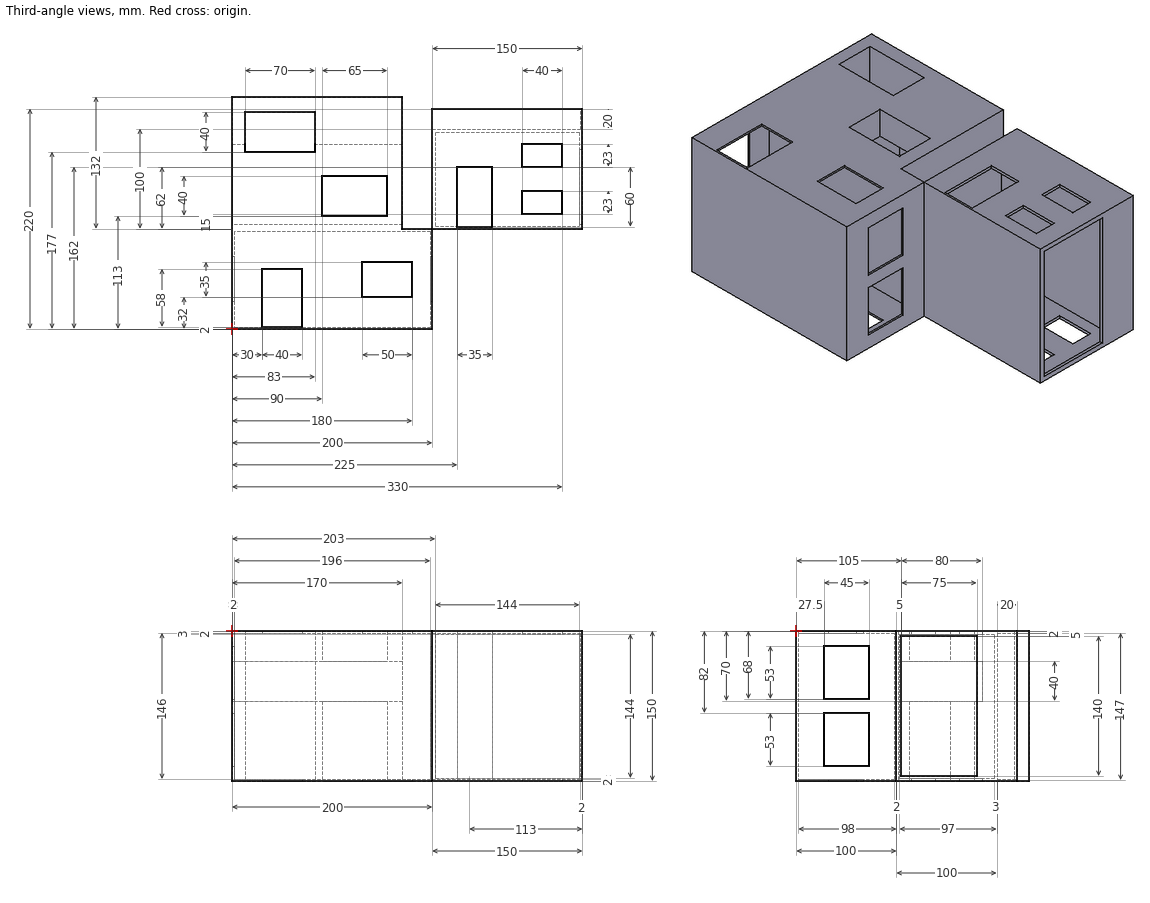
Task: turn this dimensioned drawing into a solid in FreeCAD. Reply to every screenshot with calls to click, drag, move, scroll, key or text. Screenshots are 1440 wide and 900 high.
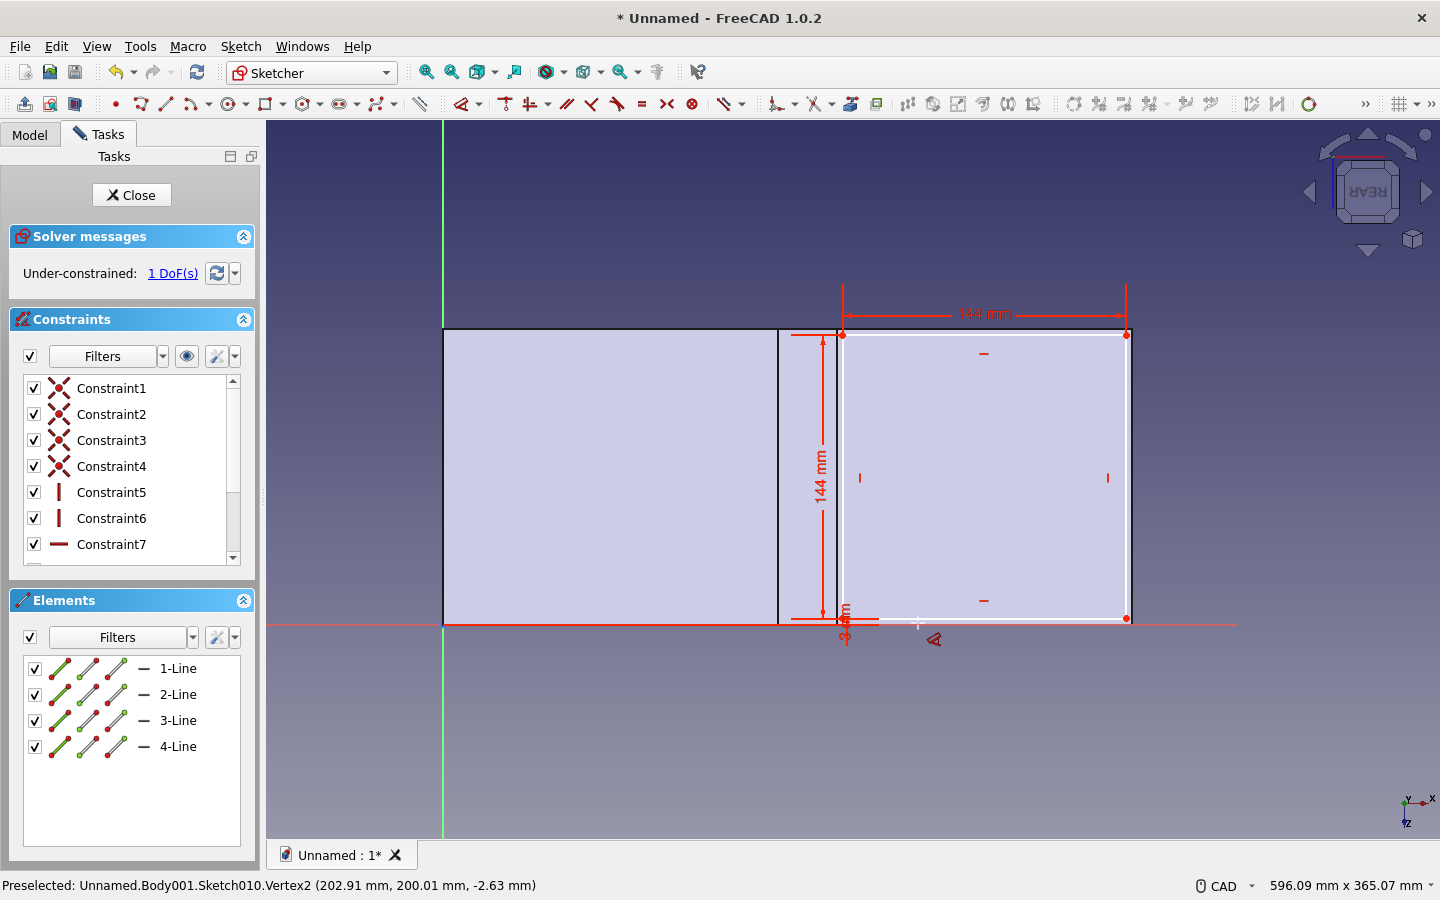
click(843, 335)
click(643, 659)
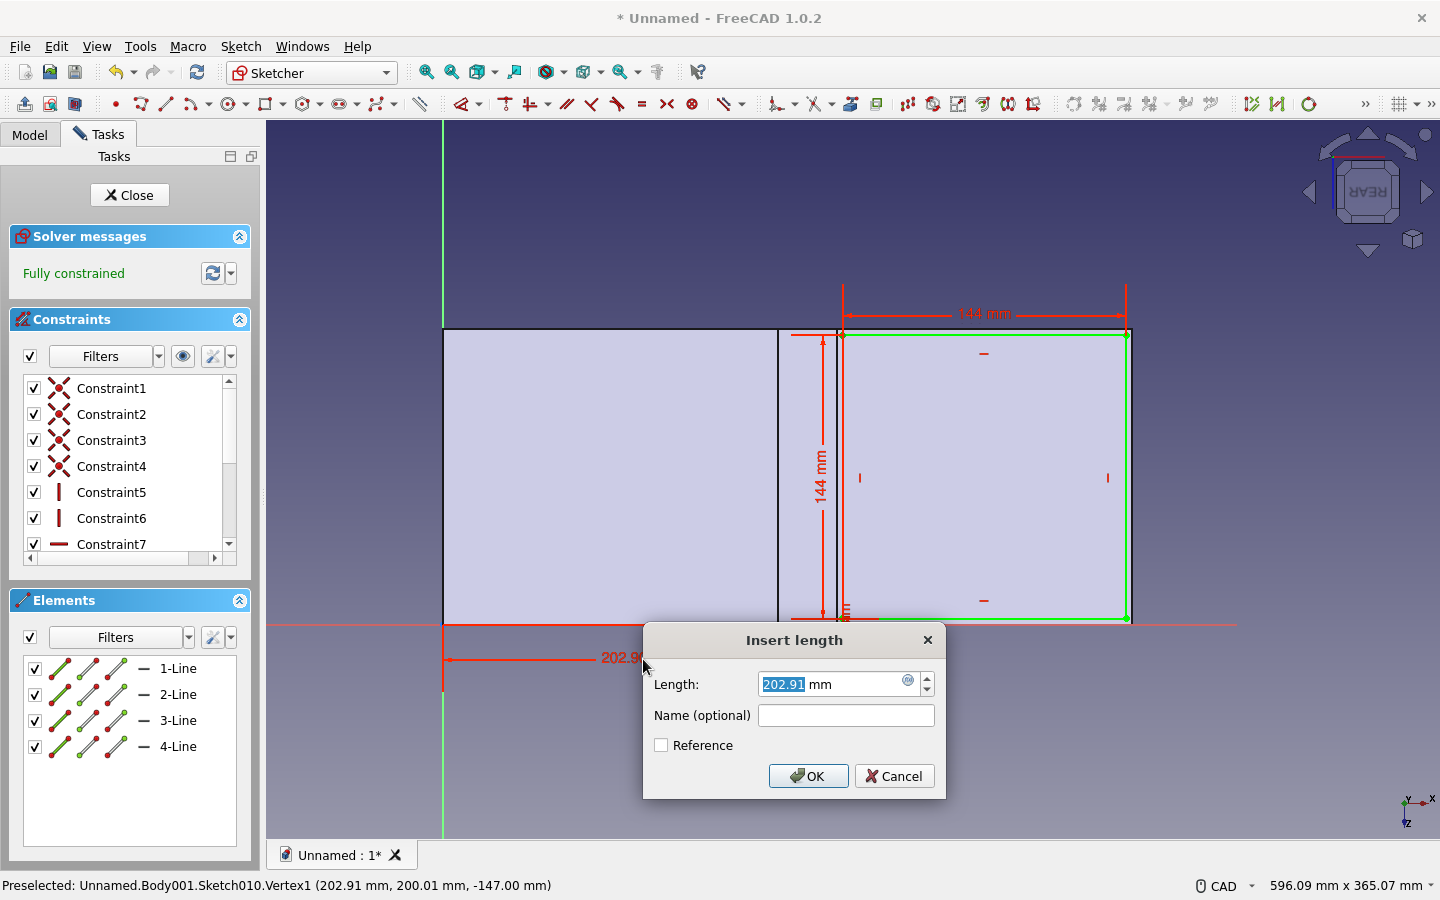
text(203)
key(Return)
key(Escape)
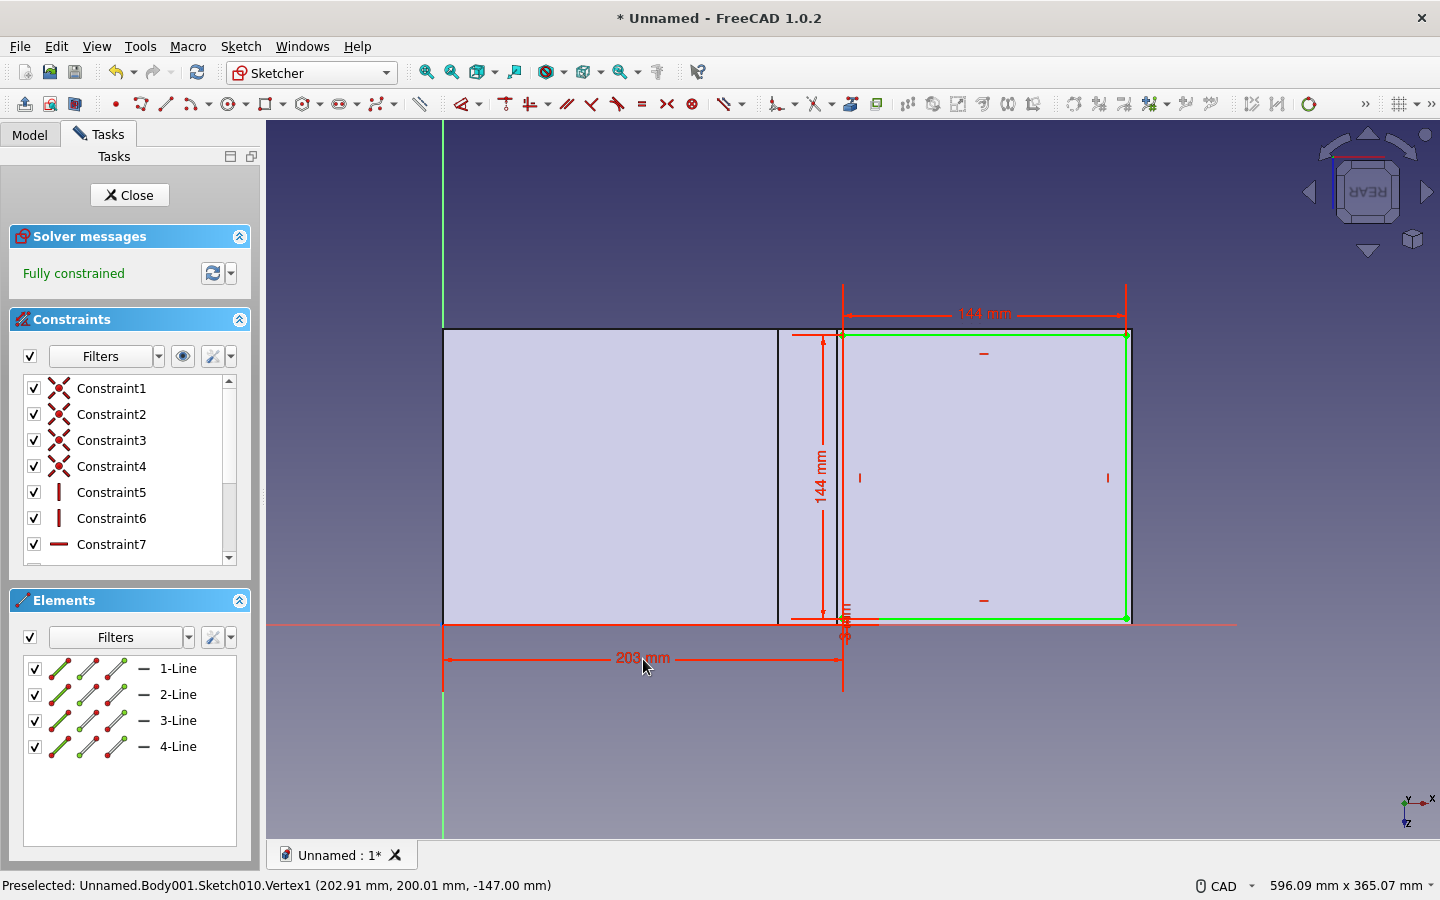
click(130, 195)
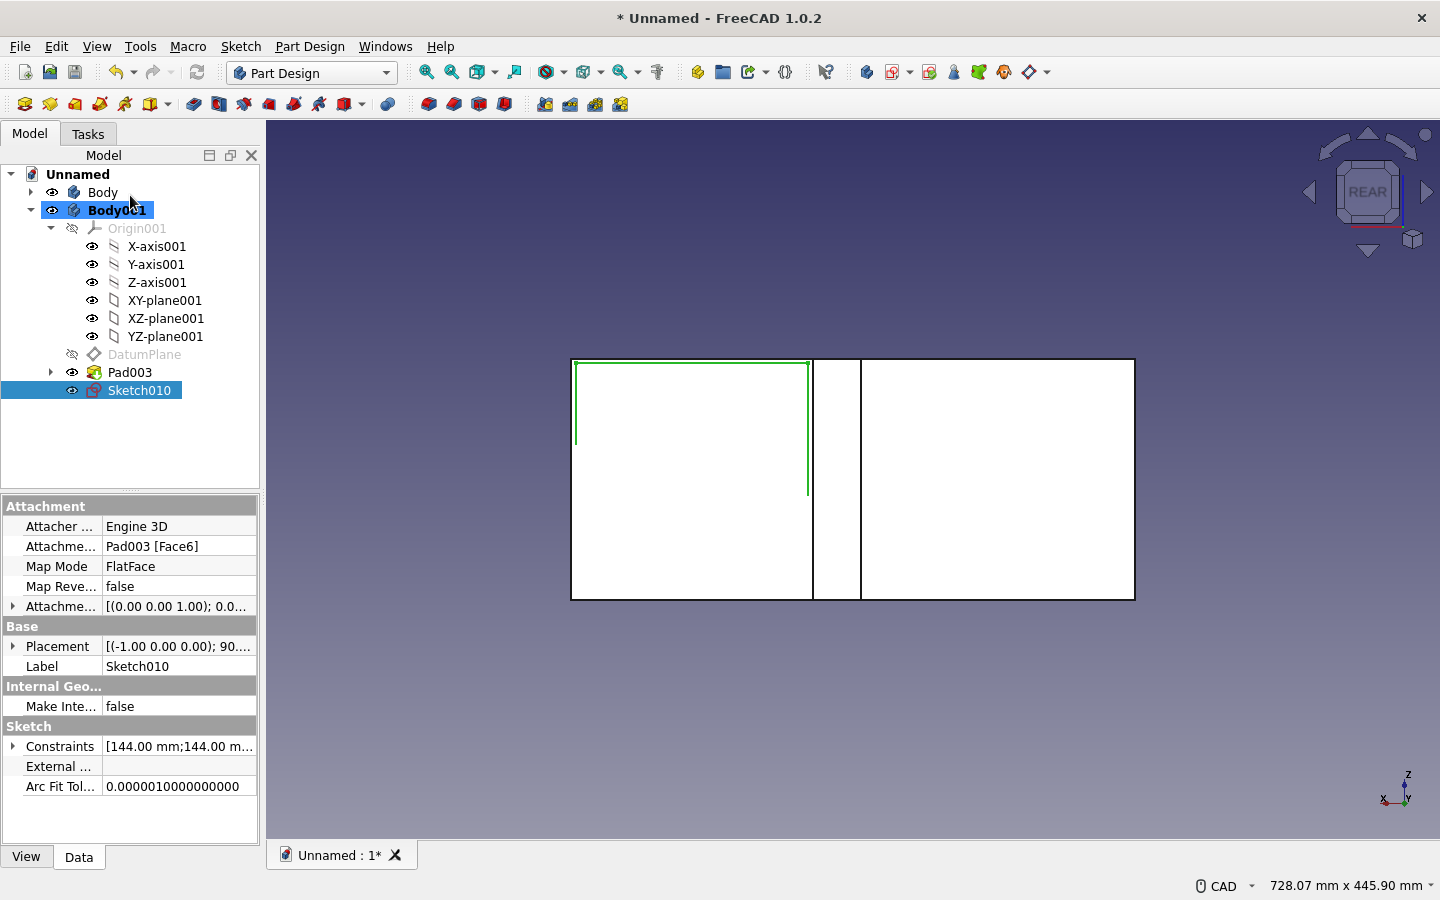
click(194, 104)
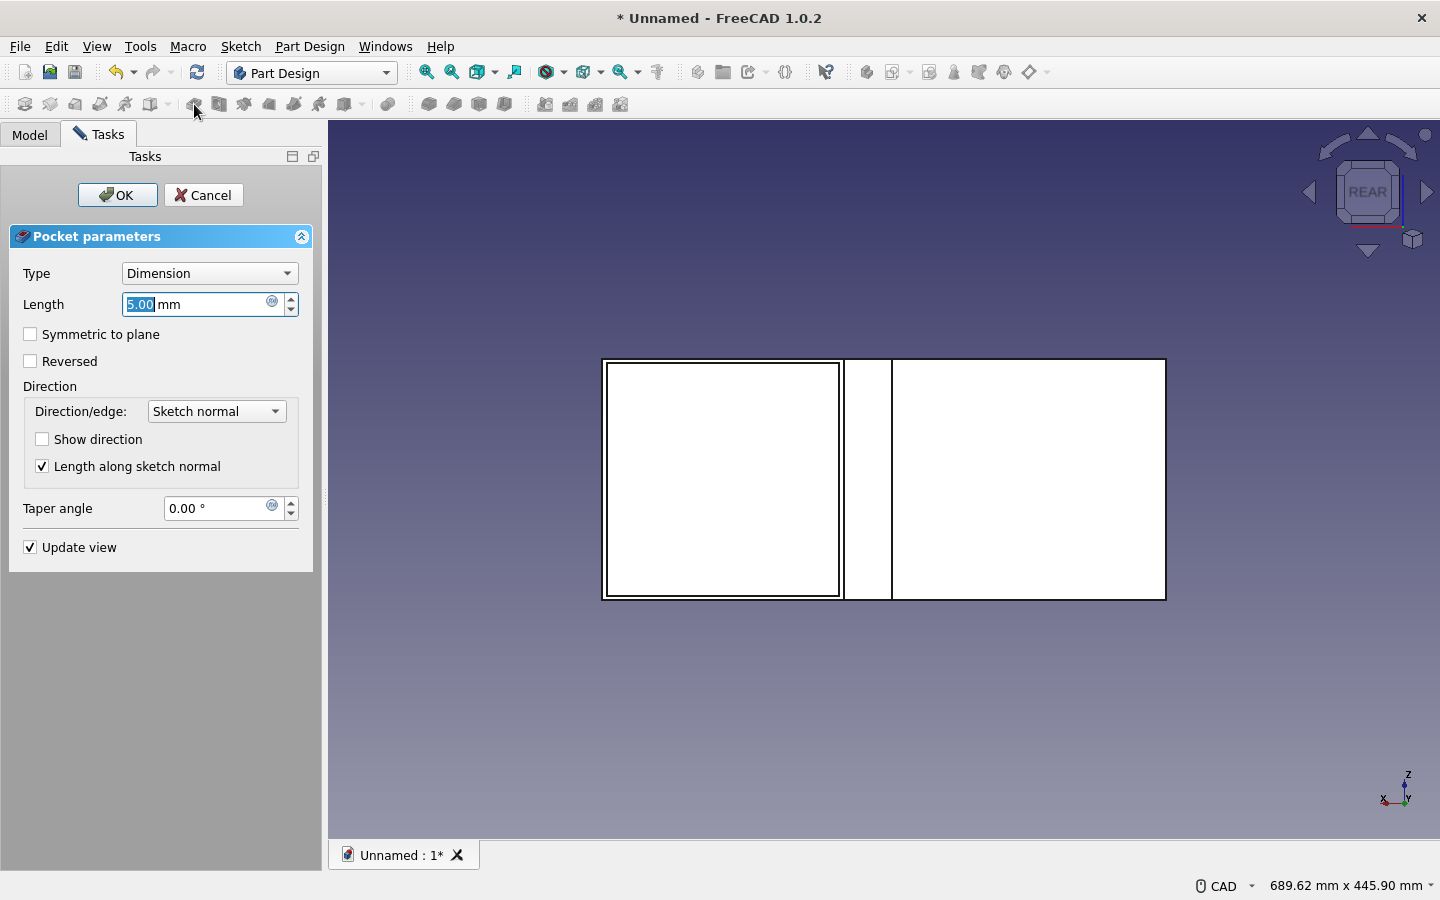
text(97)
key(Tab)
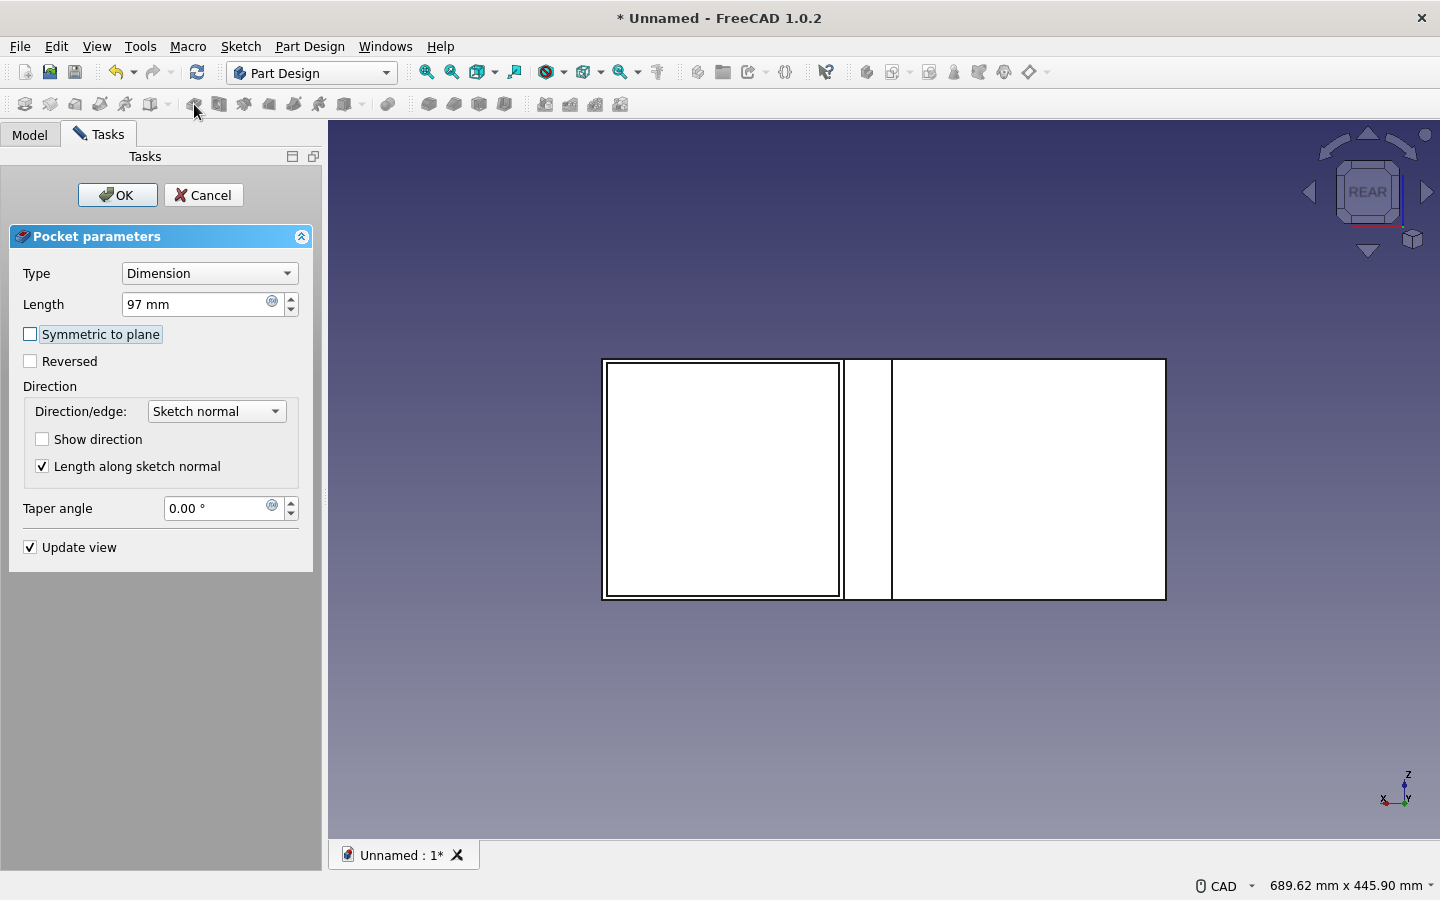
click(118, 195)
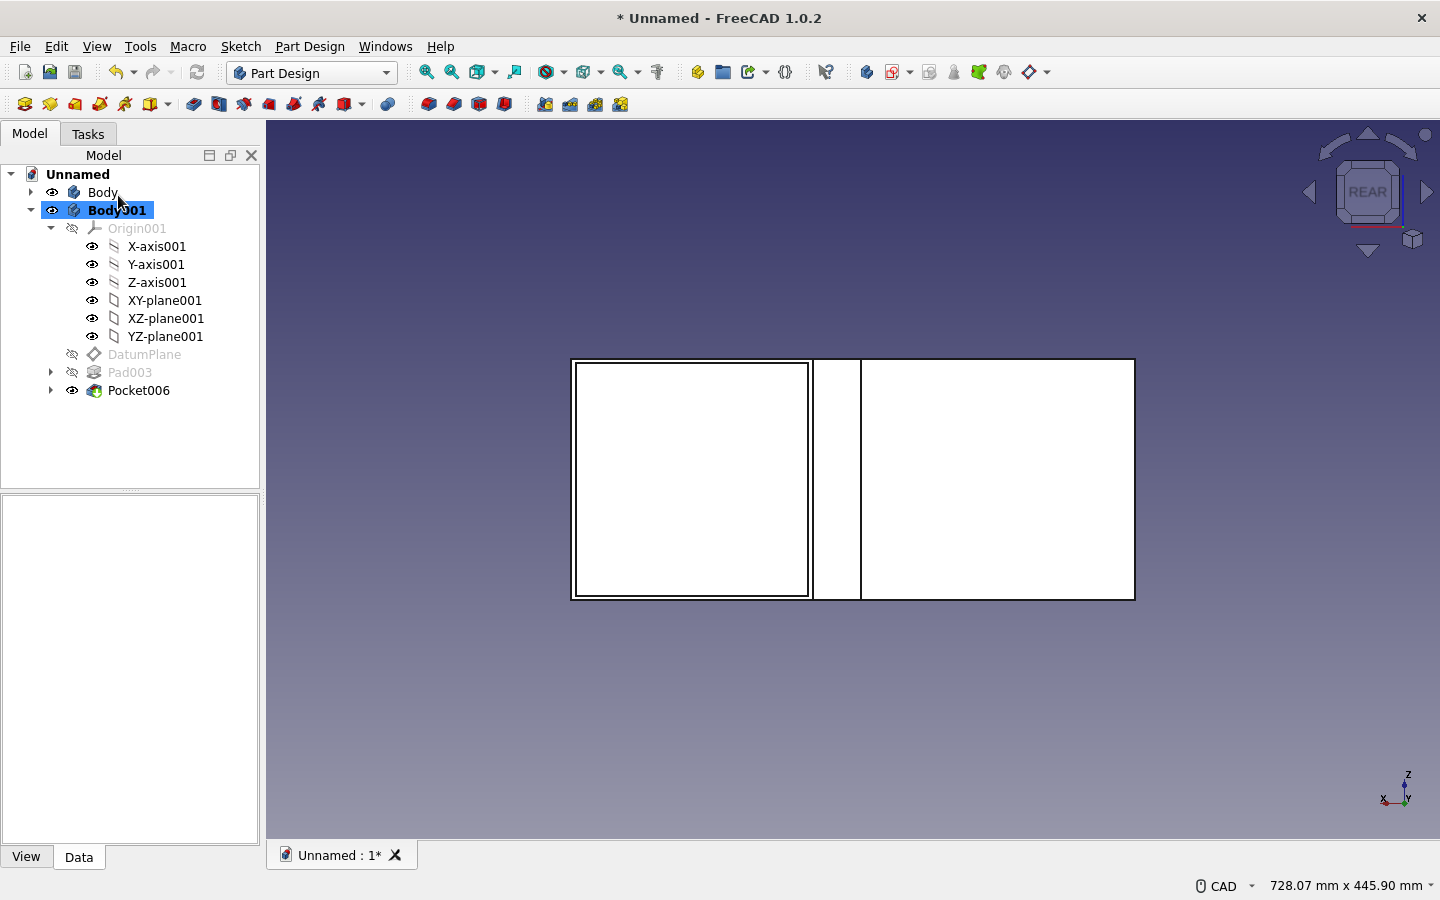
click(427, 72)